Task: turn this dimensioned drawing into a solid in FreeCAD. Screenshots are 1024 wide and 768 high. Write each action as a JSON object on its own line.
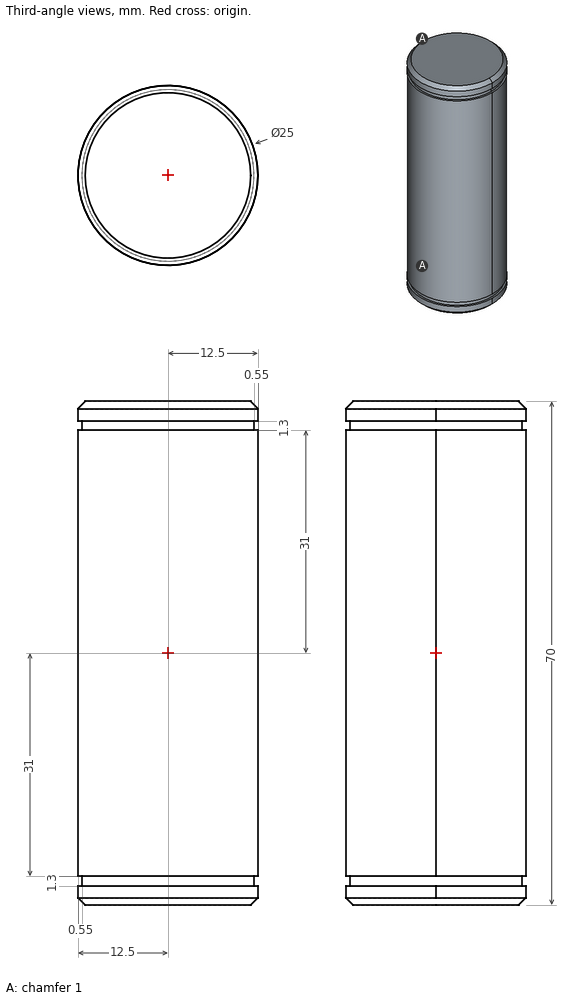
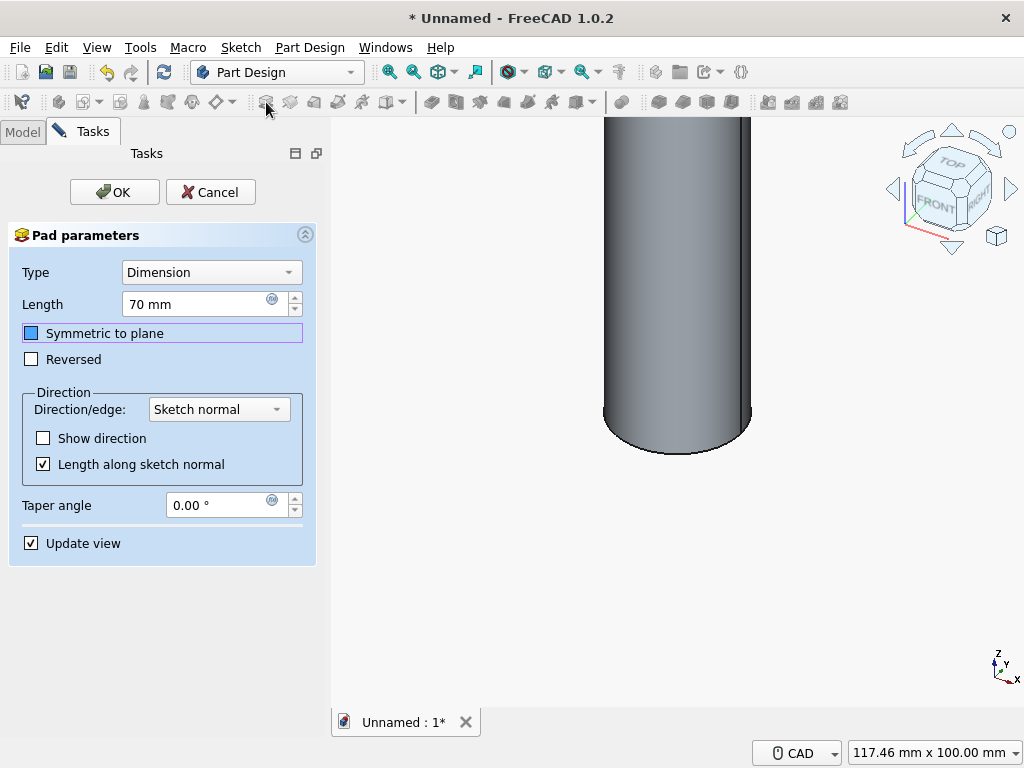
{"action": "left_click", "coordinate": [30, 333]}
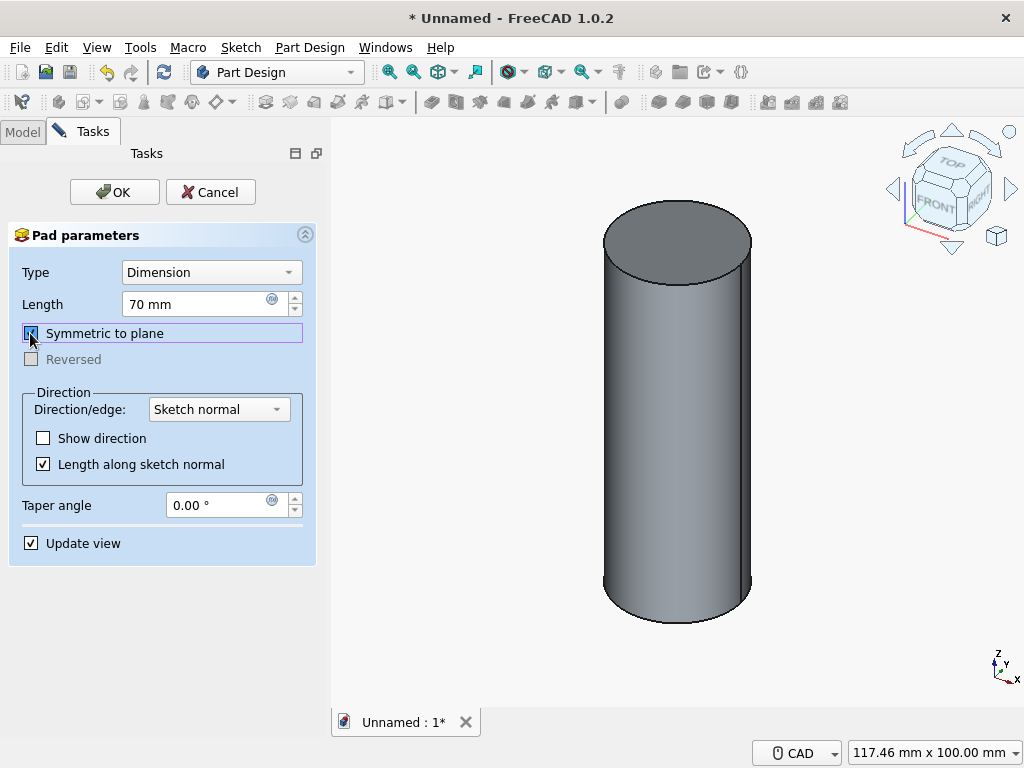
{"action": "left_click", "coordinate": [115, 192]}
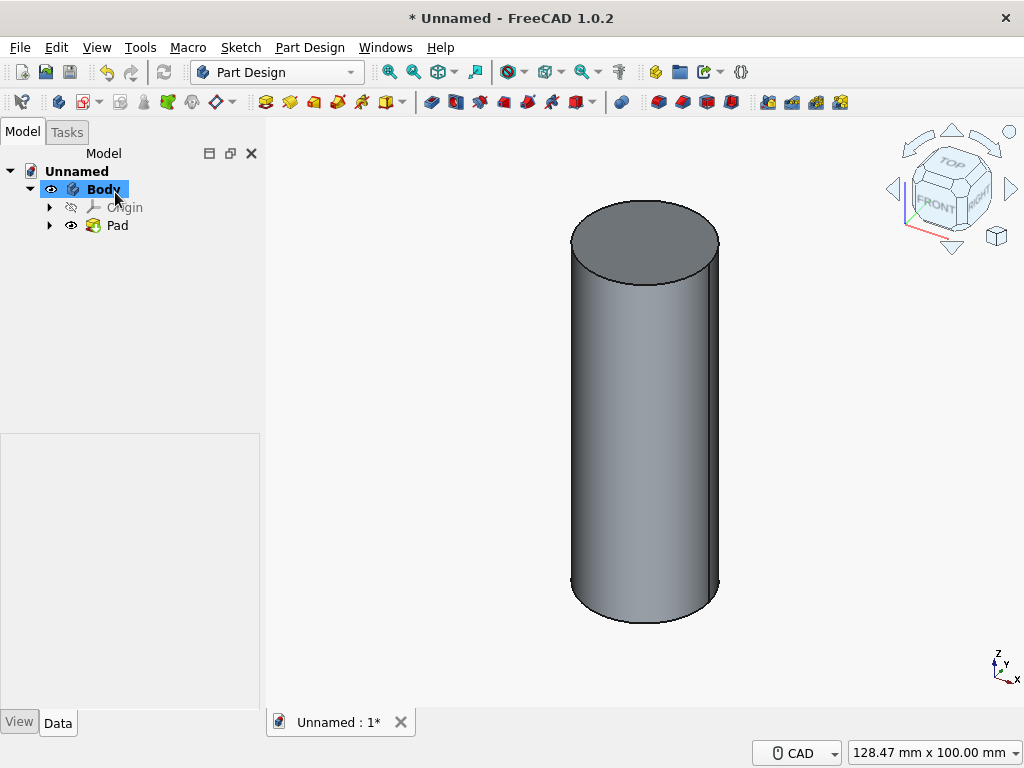
{"action": "left_click", "coordinate": [84, 102]}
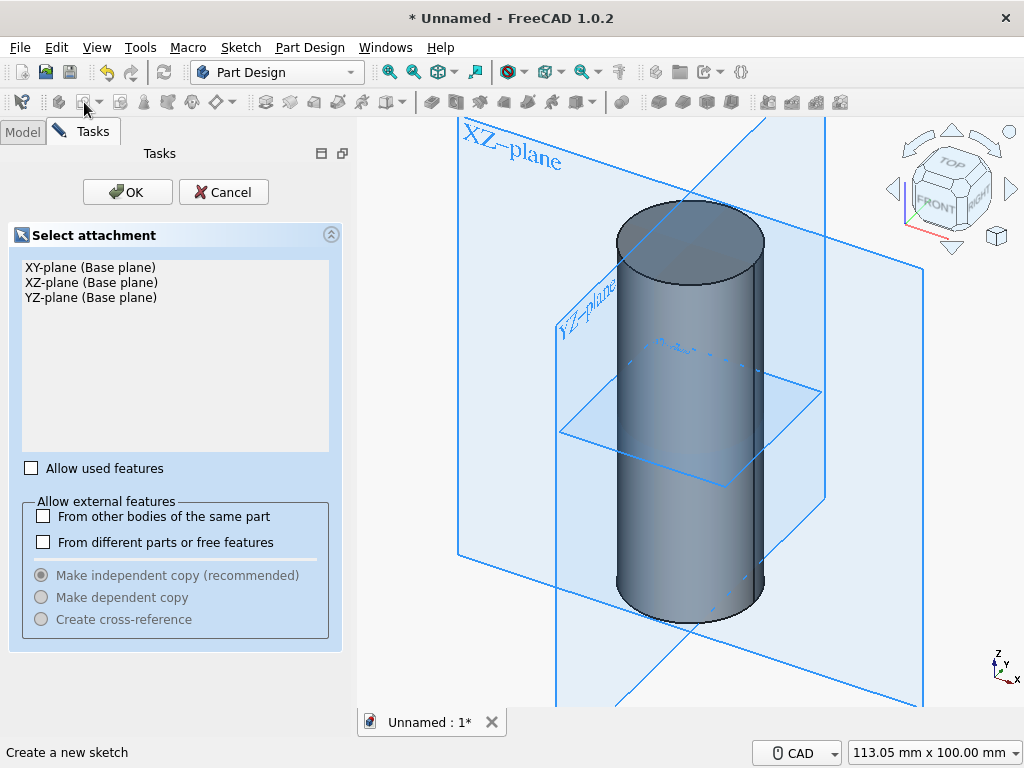
{"action": "left_click", "coordinate": [82, 282]}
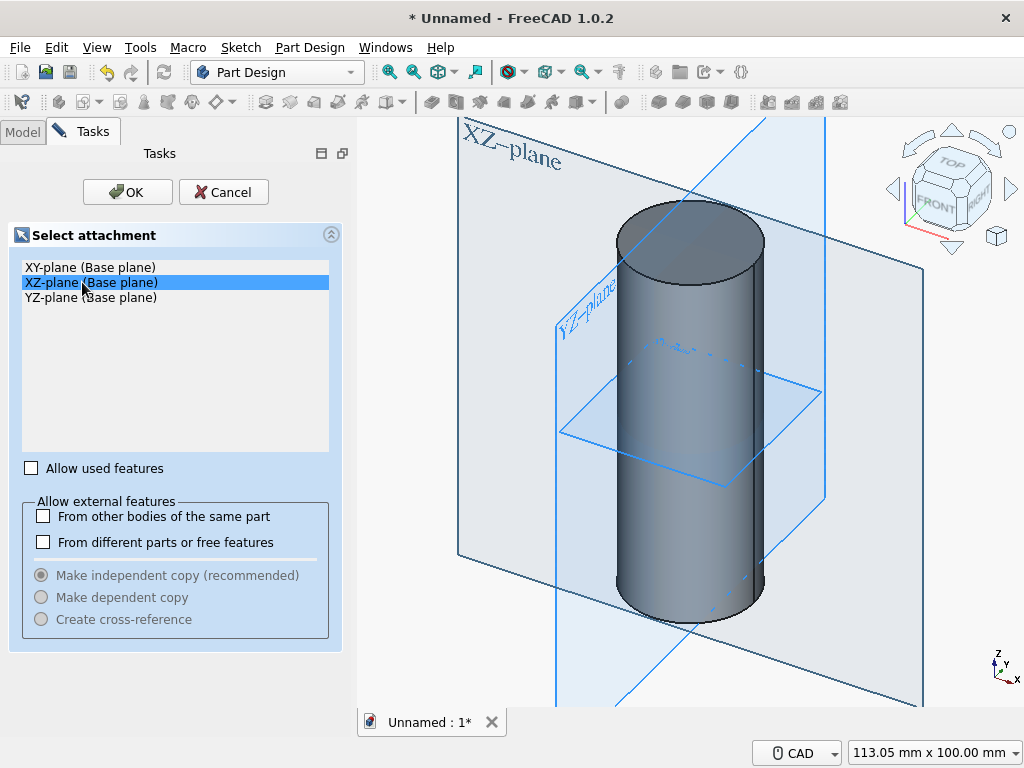
{"action": "left_click", "coordinate": [128, 192]}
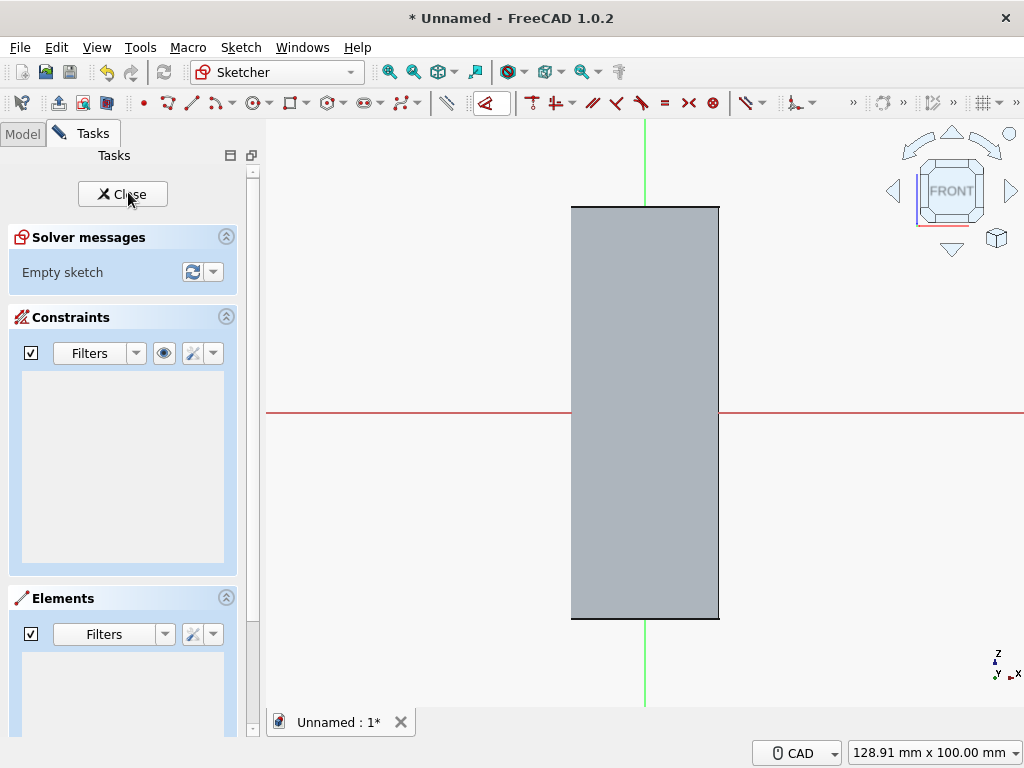
{"action": "key", "text": "q s"}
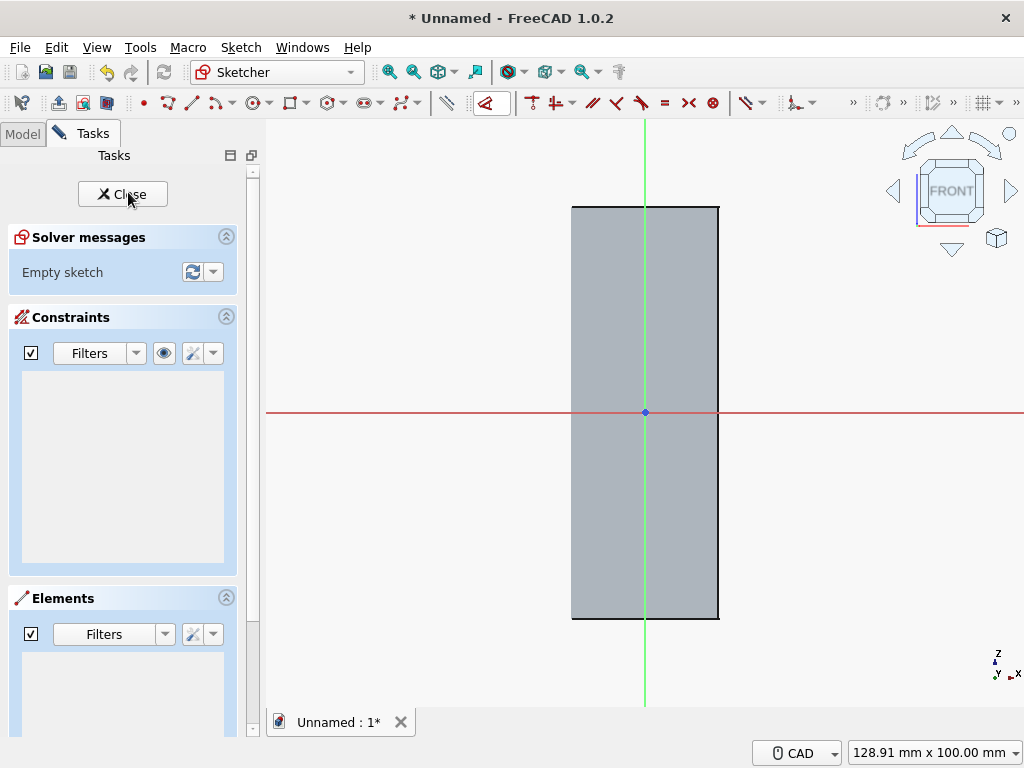
{"action": "scroll", "coordinate": [573, 609], "scroll_direction": "up", "scroll_amount": 15}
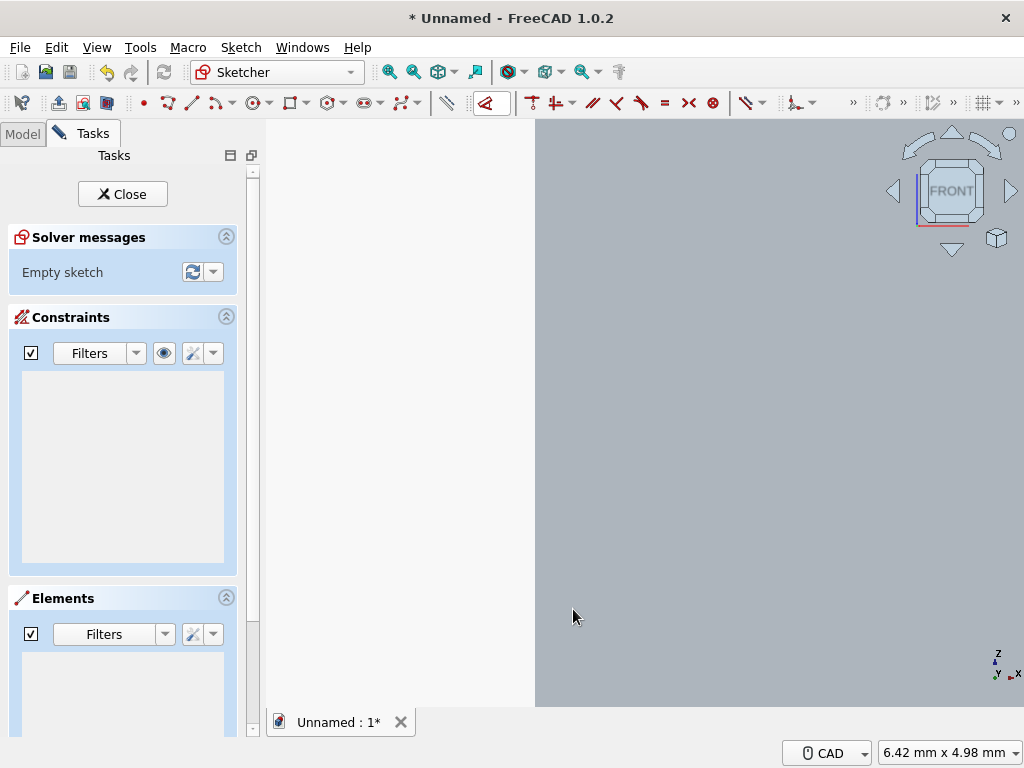
{"action": "scroll", "coordinate": [560, 379], "scroll_direction": "up", "scroll_amount": 4}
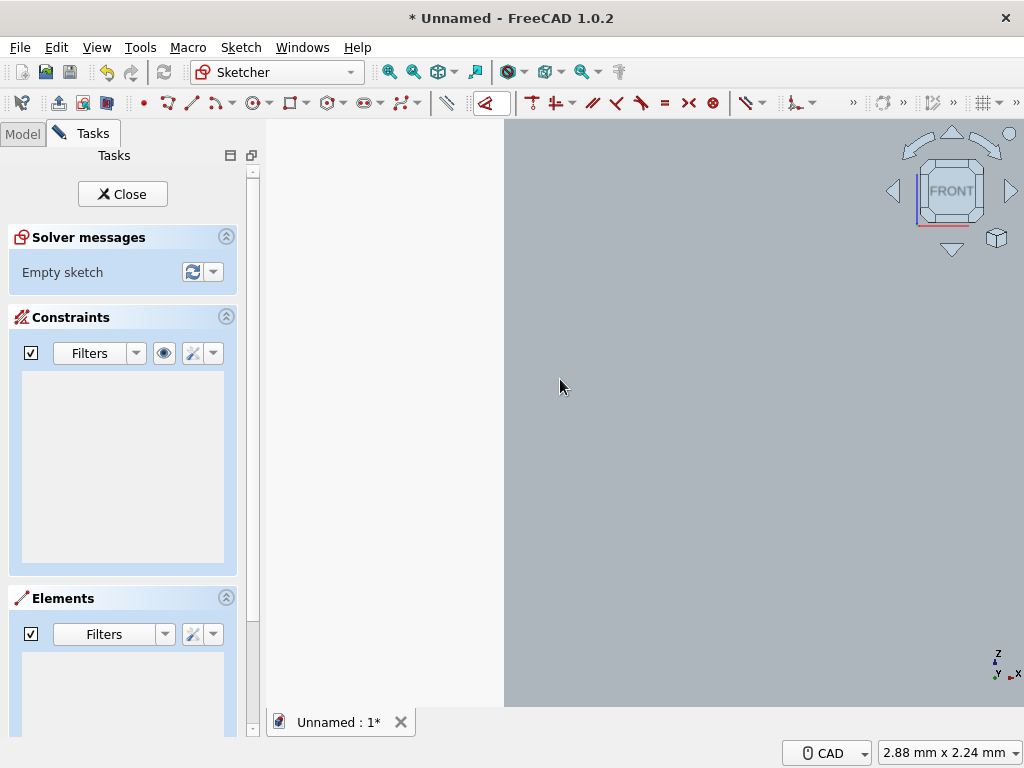
{"action": "left_click", "coordinate": [290, 104]}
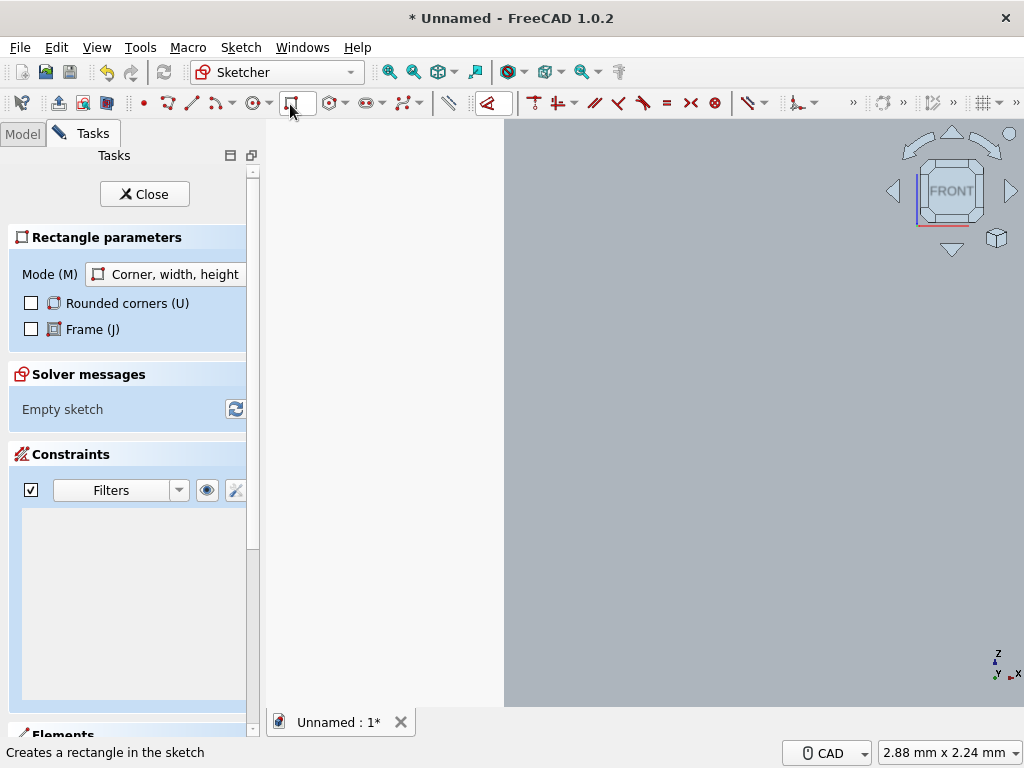
{"action": "left_click", "coordinate": [504, 242]}
{"action": "left_click", "coordinate": [649, 583]}
{"action": "key", "text": "Escape"}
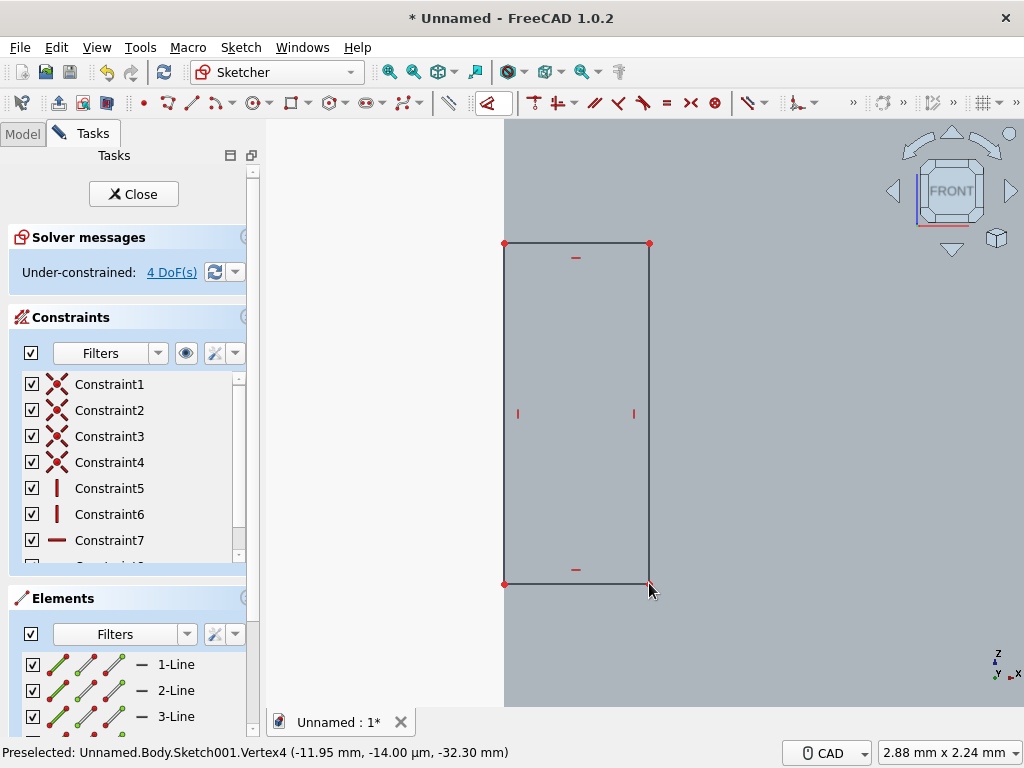
{"action": "key", "text": "d"}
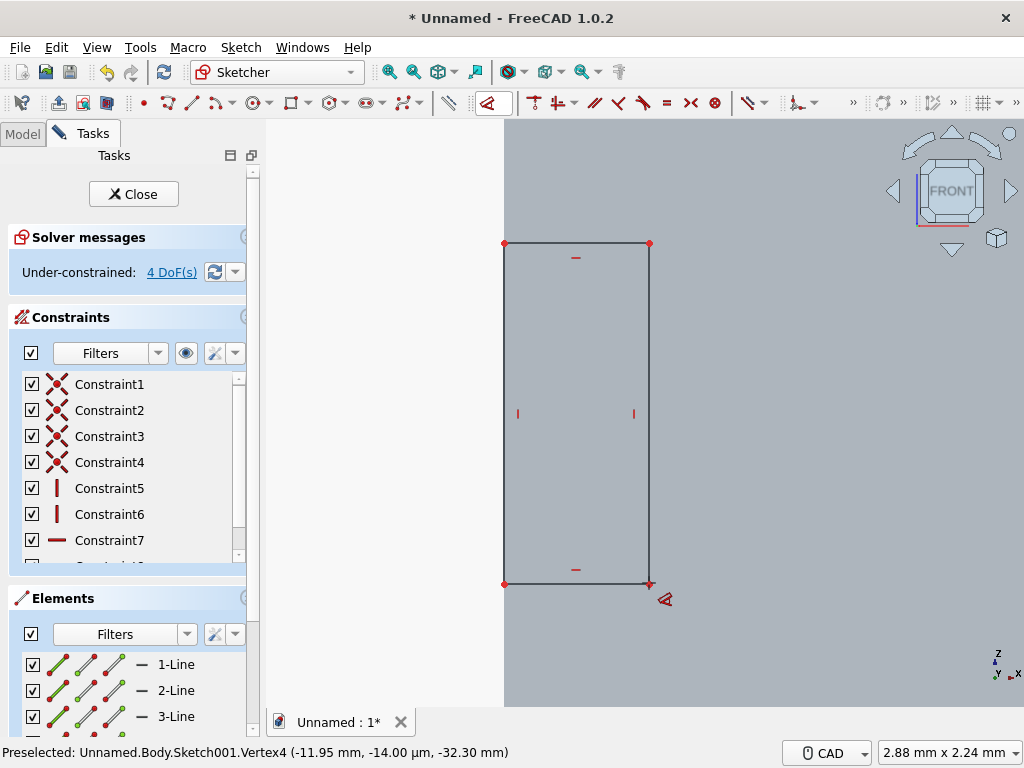
{"action": "left_click", "coordinate": [504, 345]}
{"action": "left_click", "coordinate": [470, 413]}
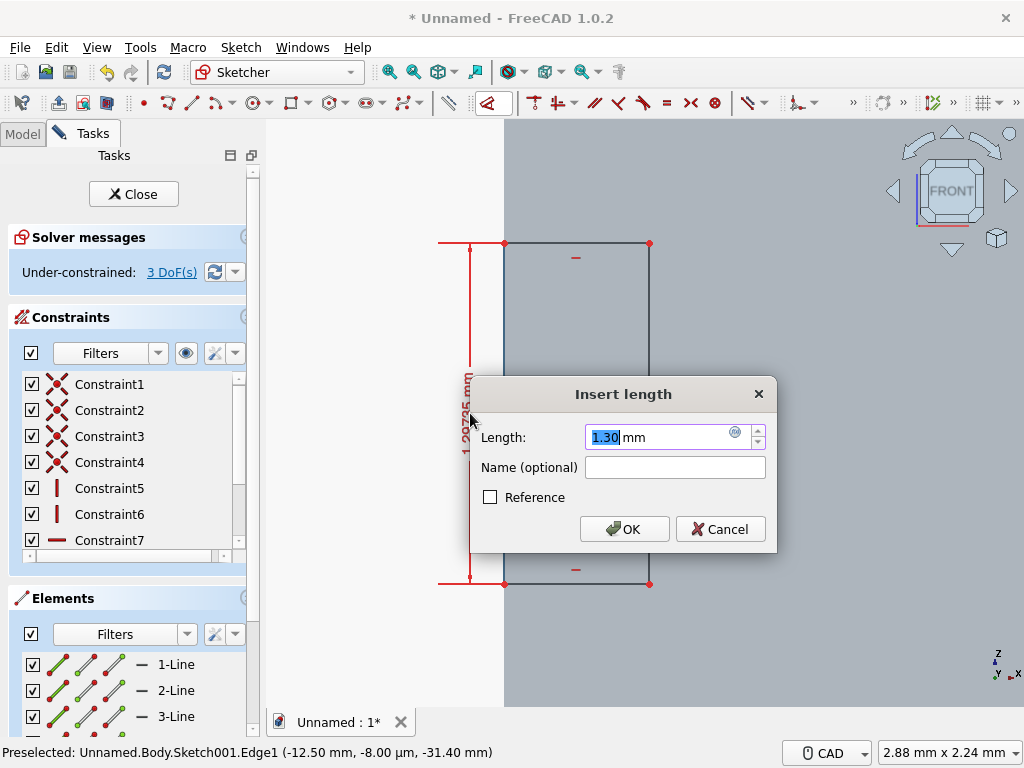
{"action": "type", "text": "1.3"}
{"action": "key", "text": "Return"}